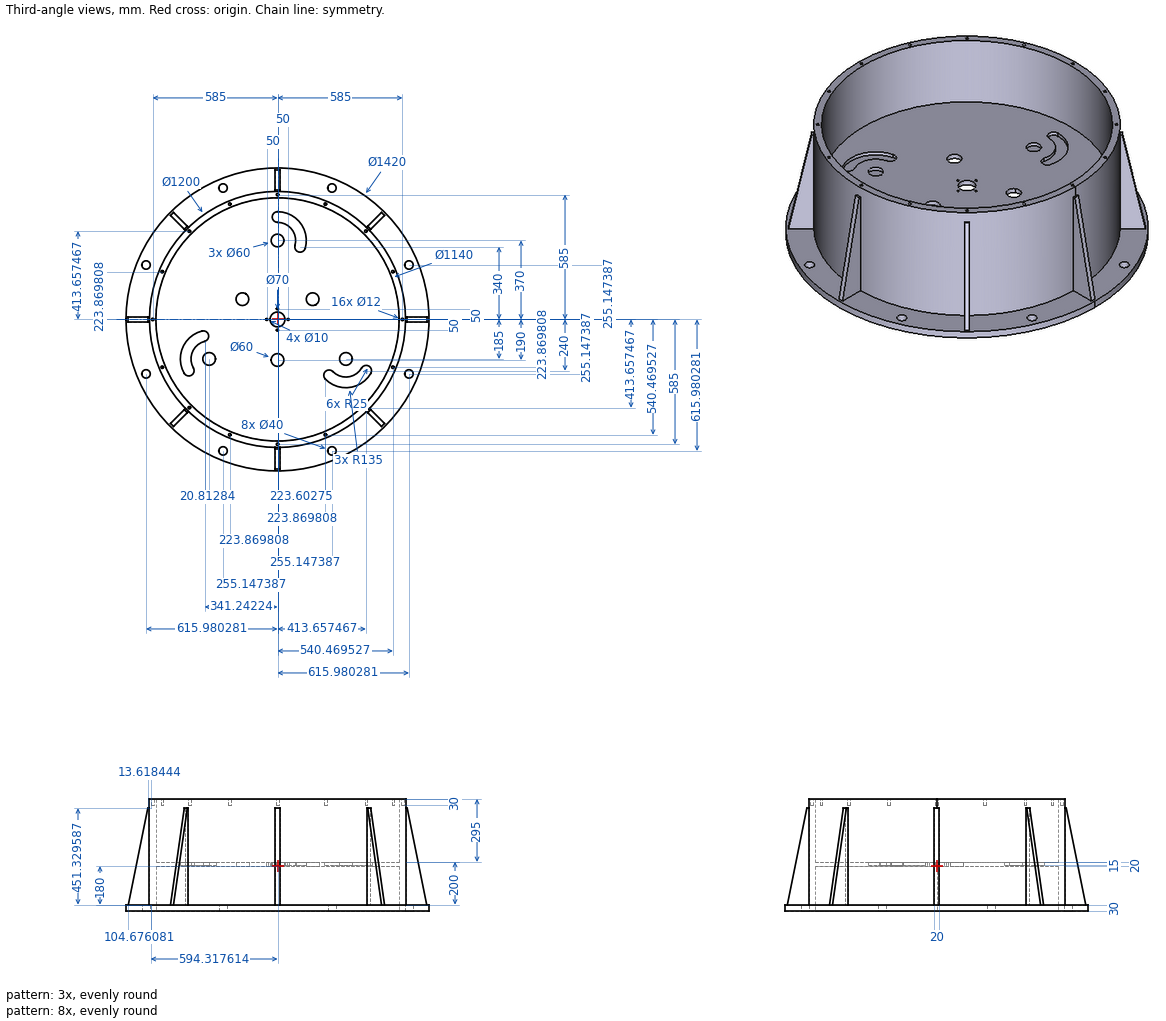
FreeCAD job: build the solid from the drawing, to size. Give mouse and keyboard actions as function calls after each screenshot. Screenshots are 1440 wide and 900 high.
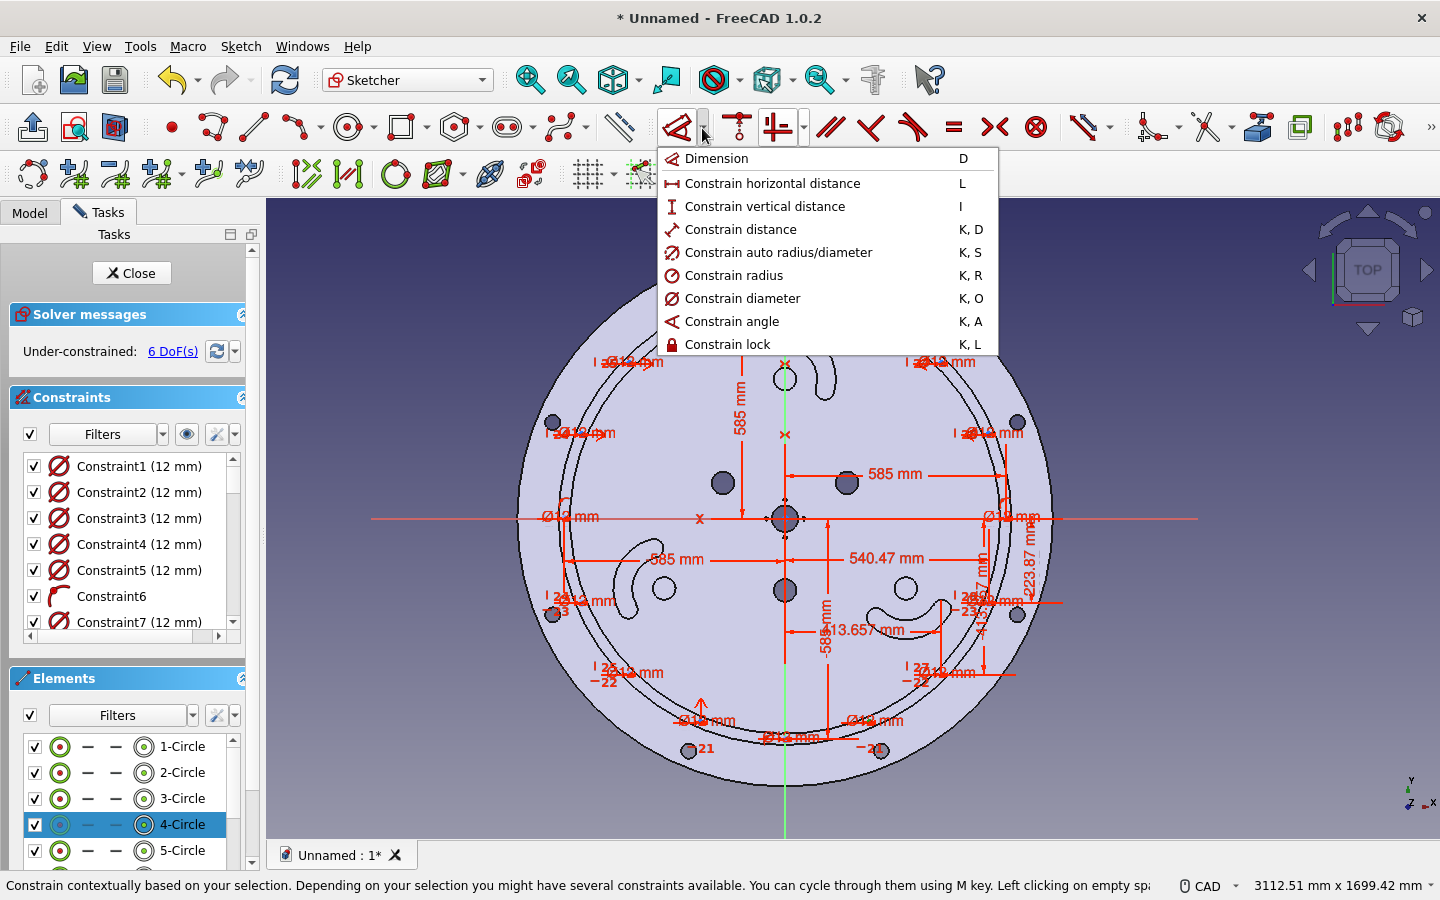
click(828, 184)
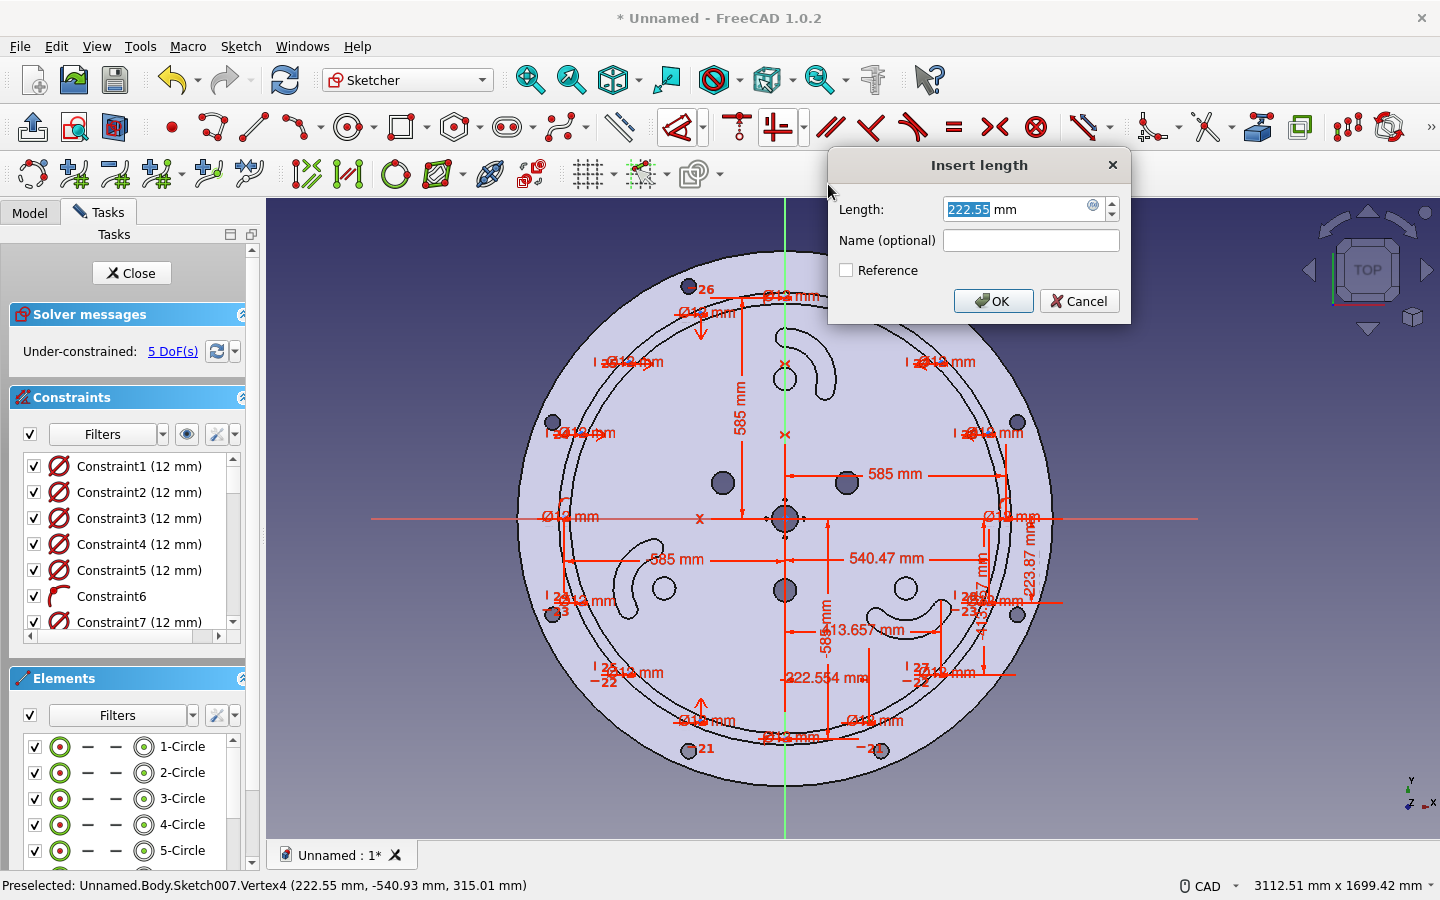
text(223.869808)
key(Return)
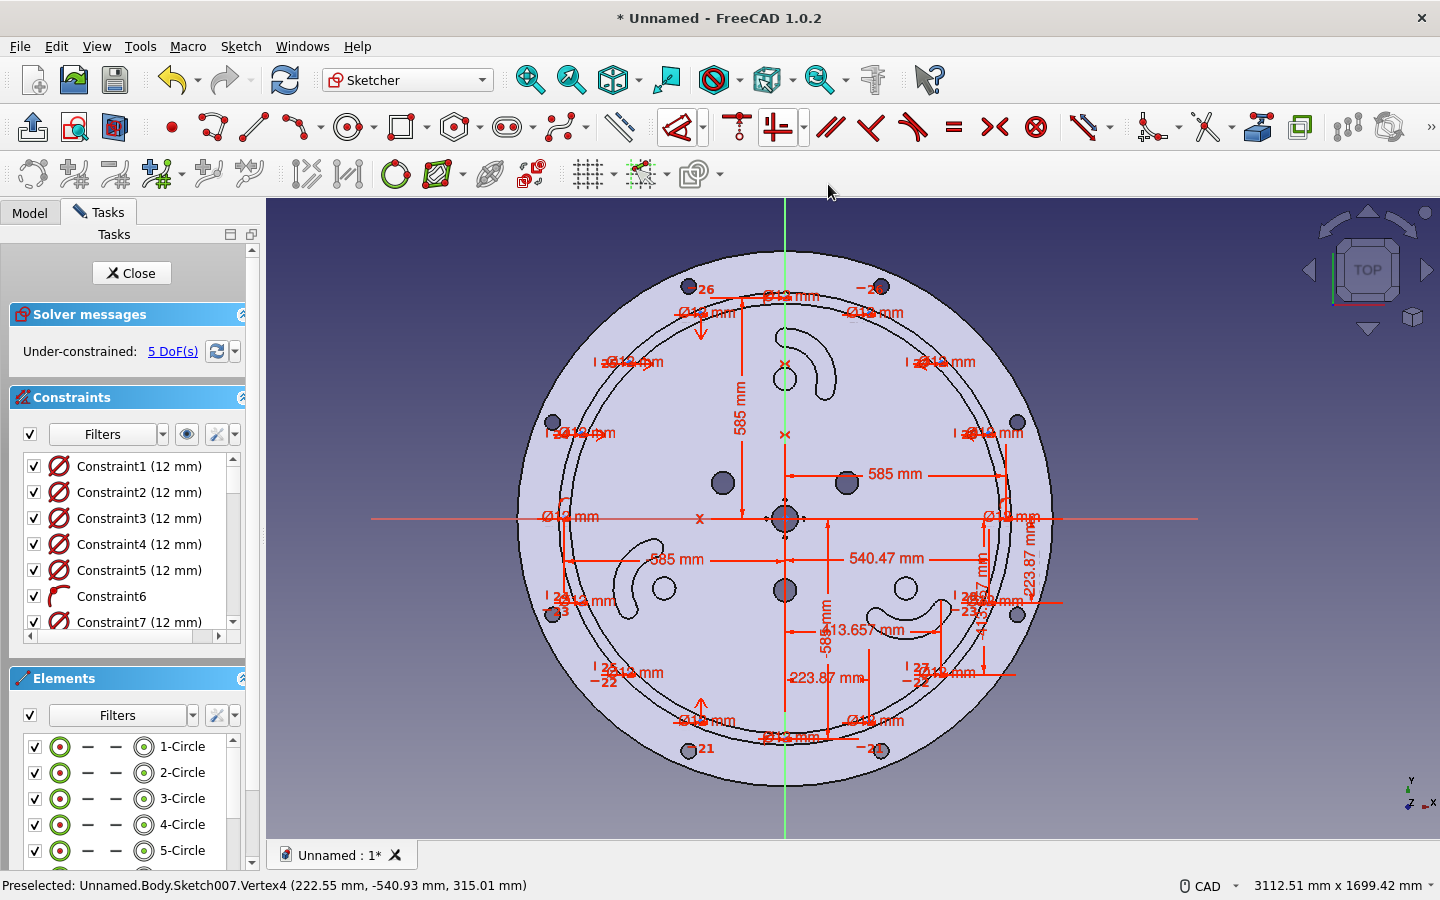
click(869, 723)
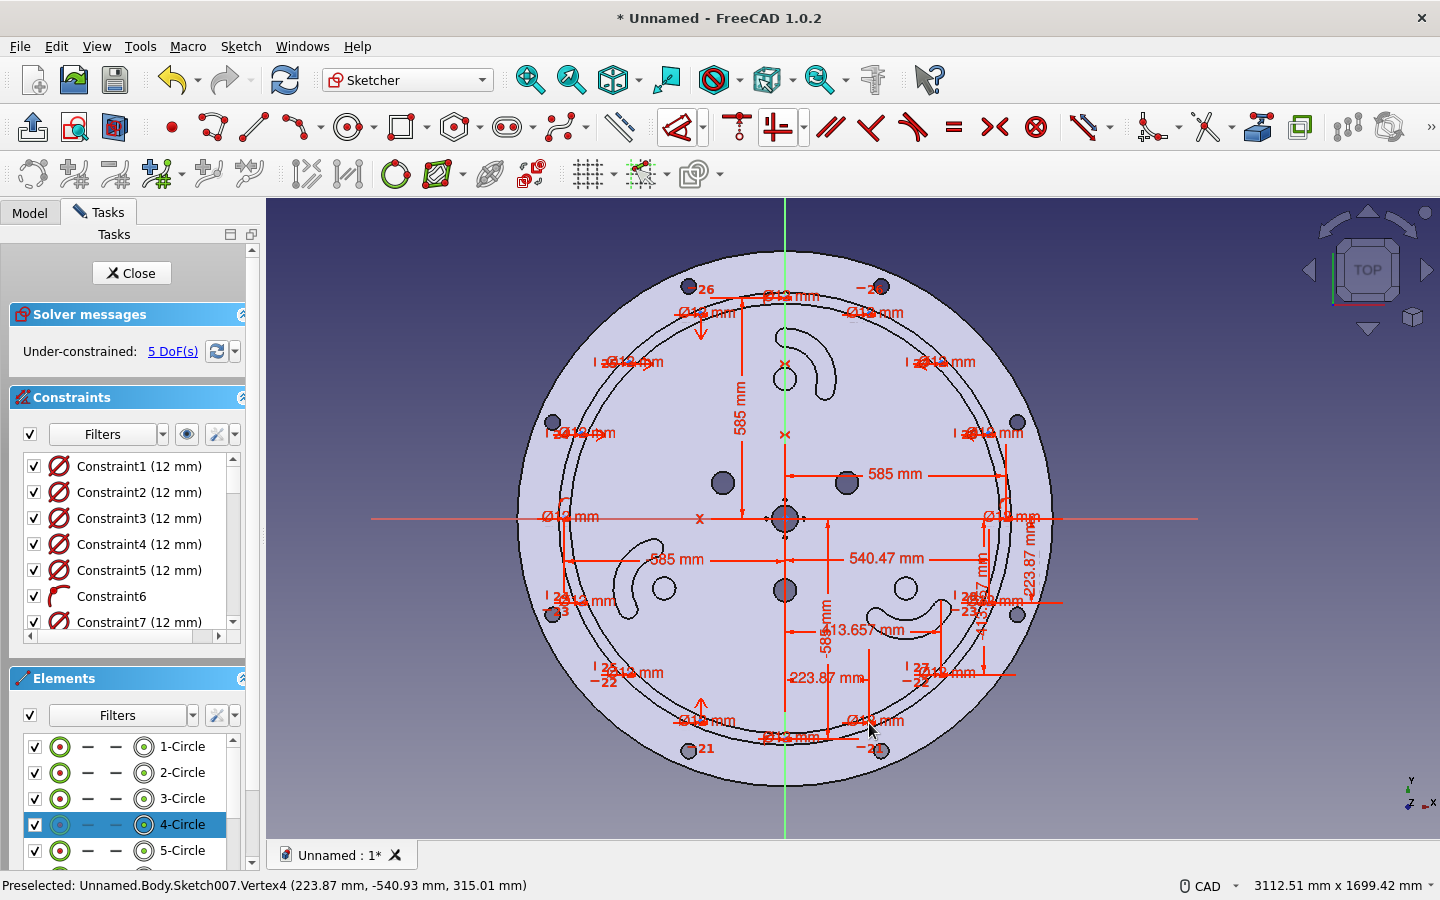
click(702, 128)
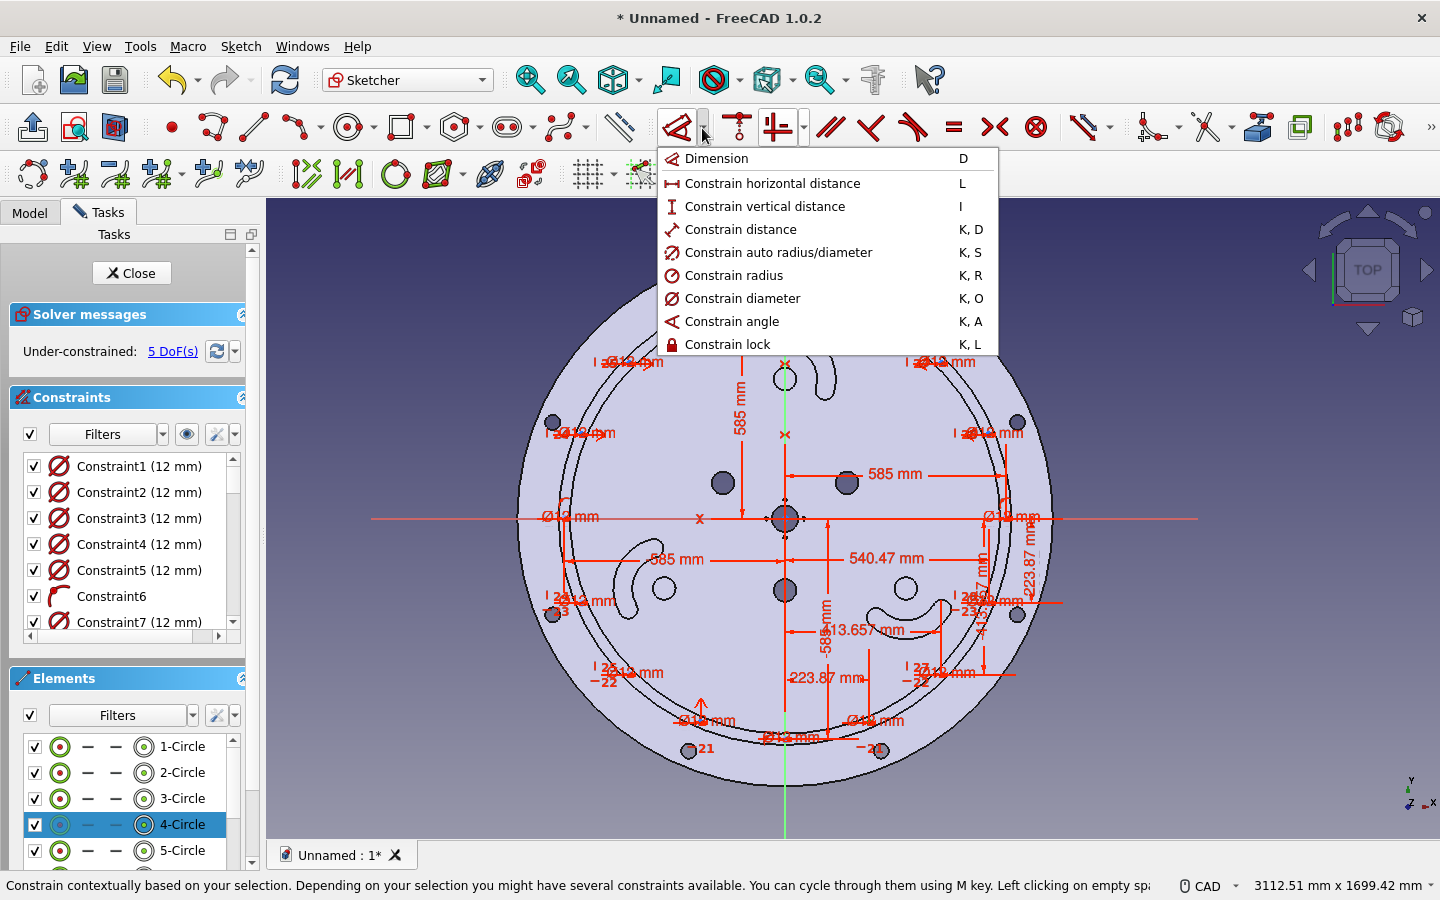
click(828, 206)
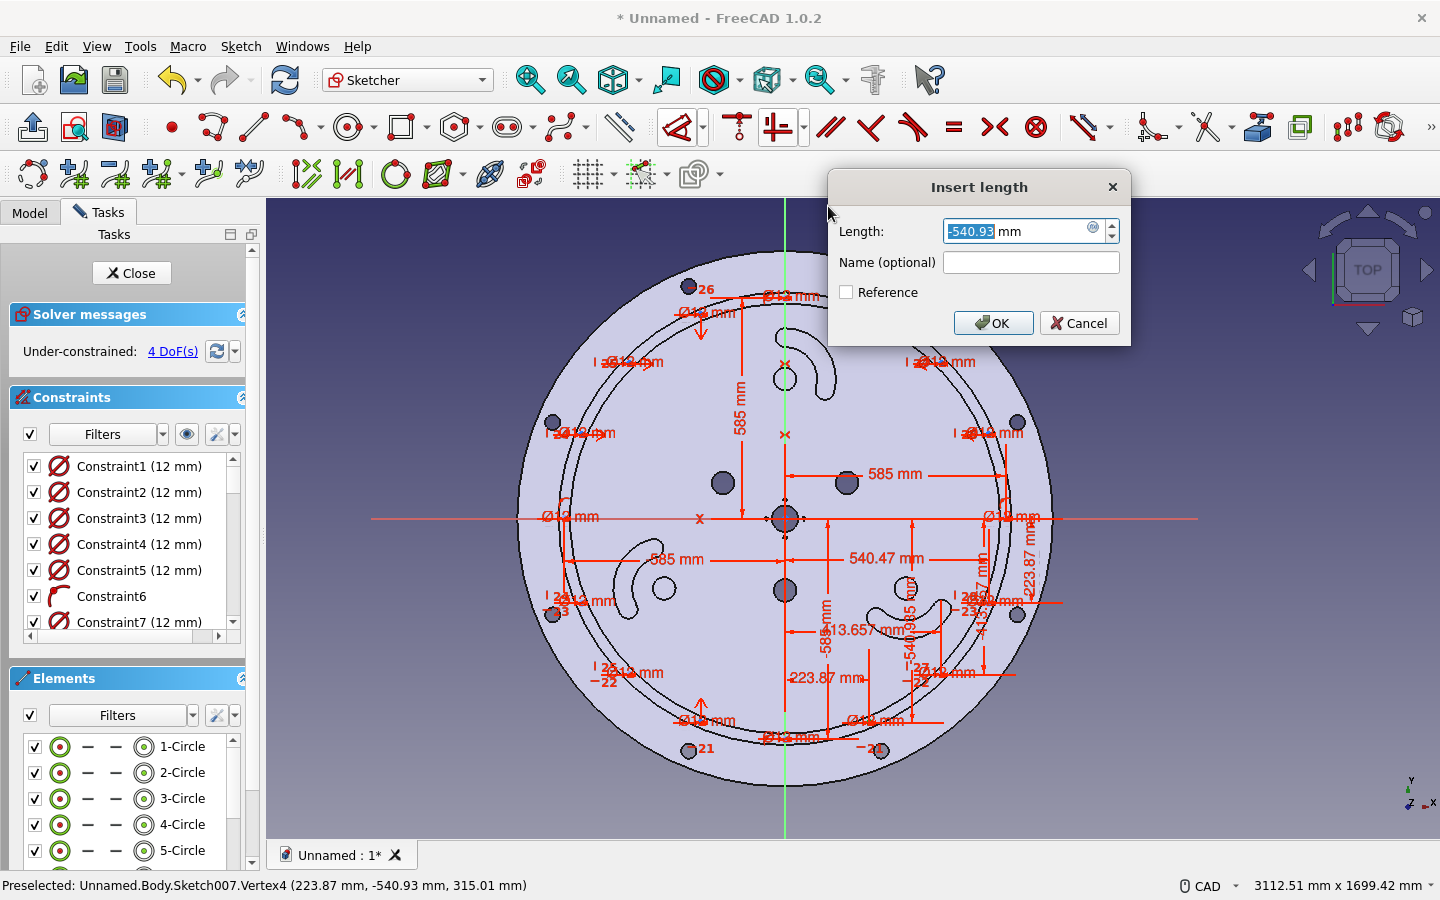
text(-540.469527)
key(Return)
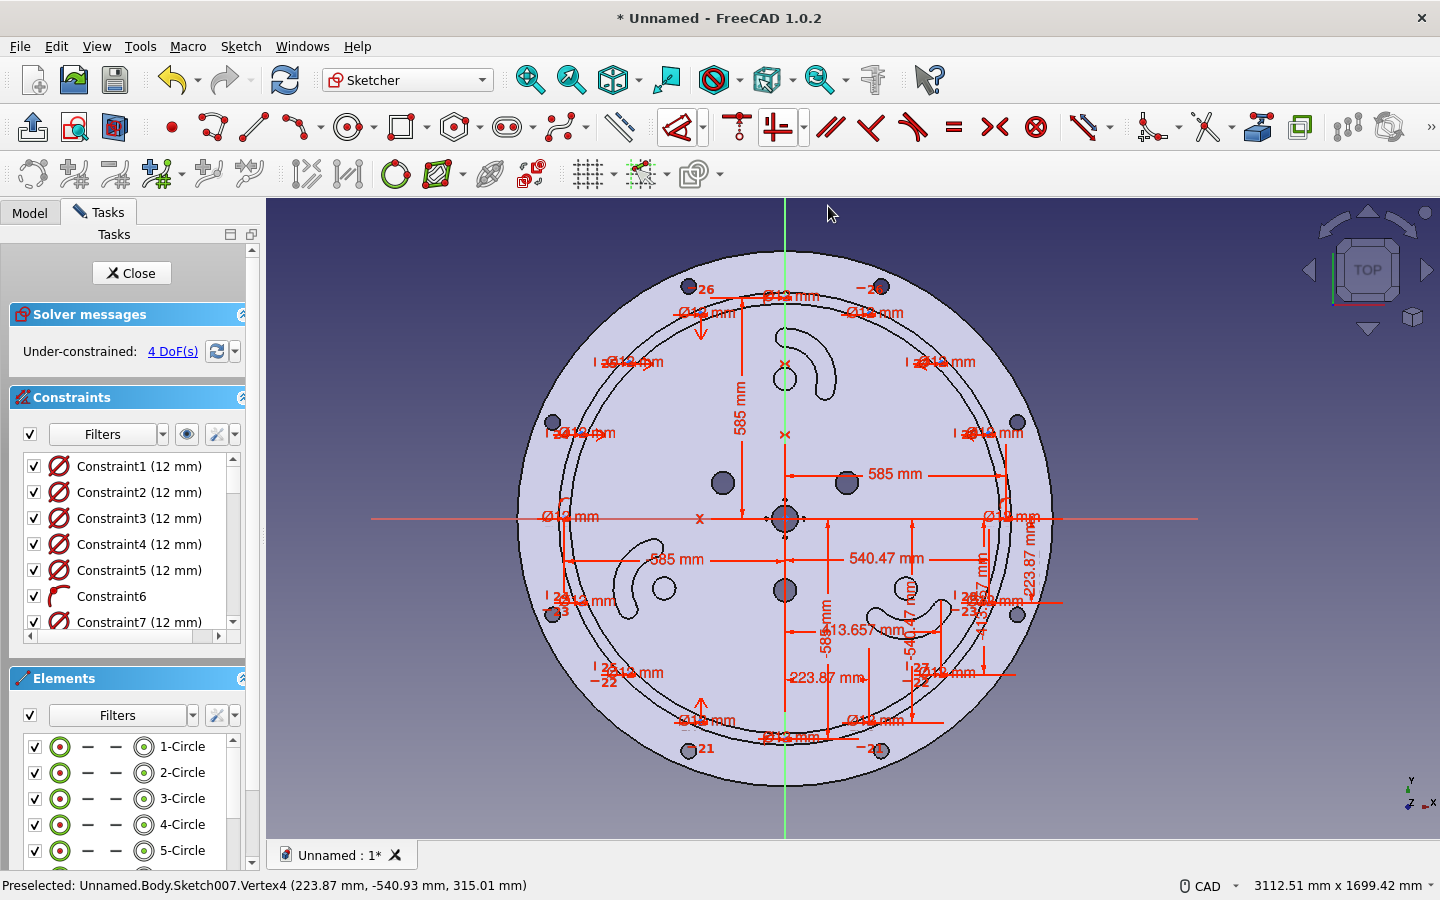
click(701, 723)